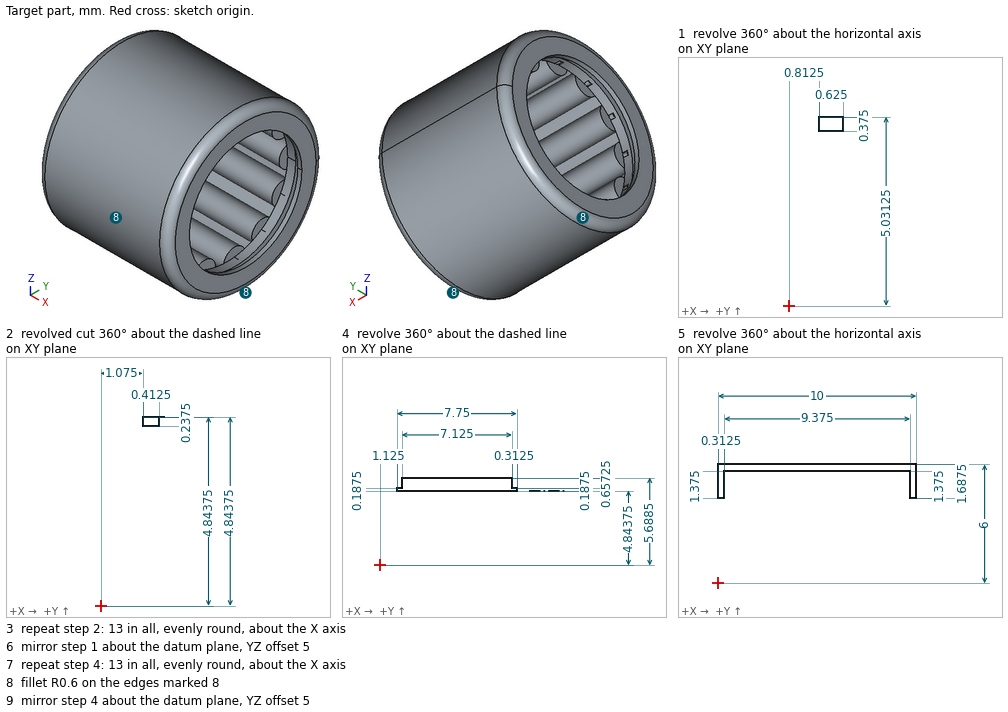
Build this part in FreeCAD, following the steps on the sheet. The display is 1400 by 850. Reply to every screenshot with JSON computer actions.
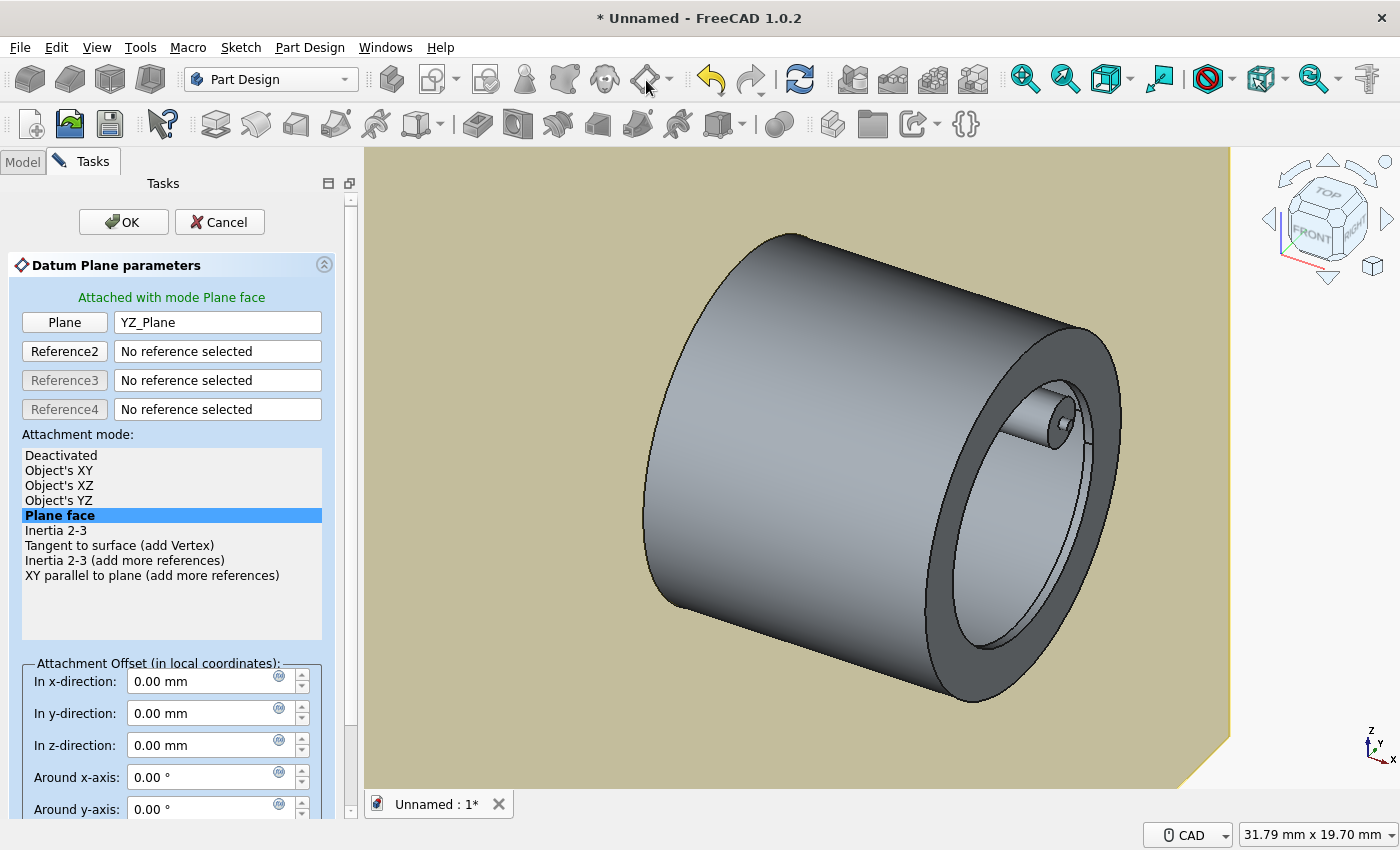
{"action": "triple_click", "coordinate": [210, 745]}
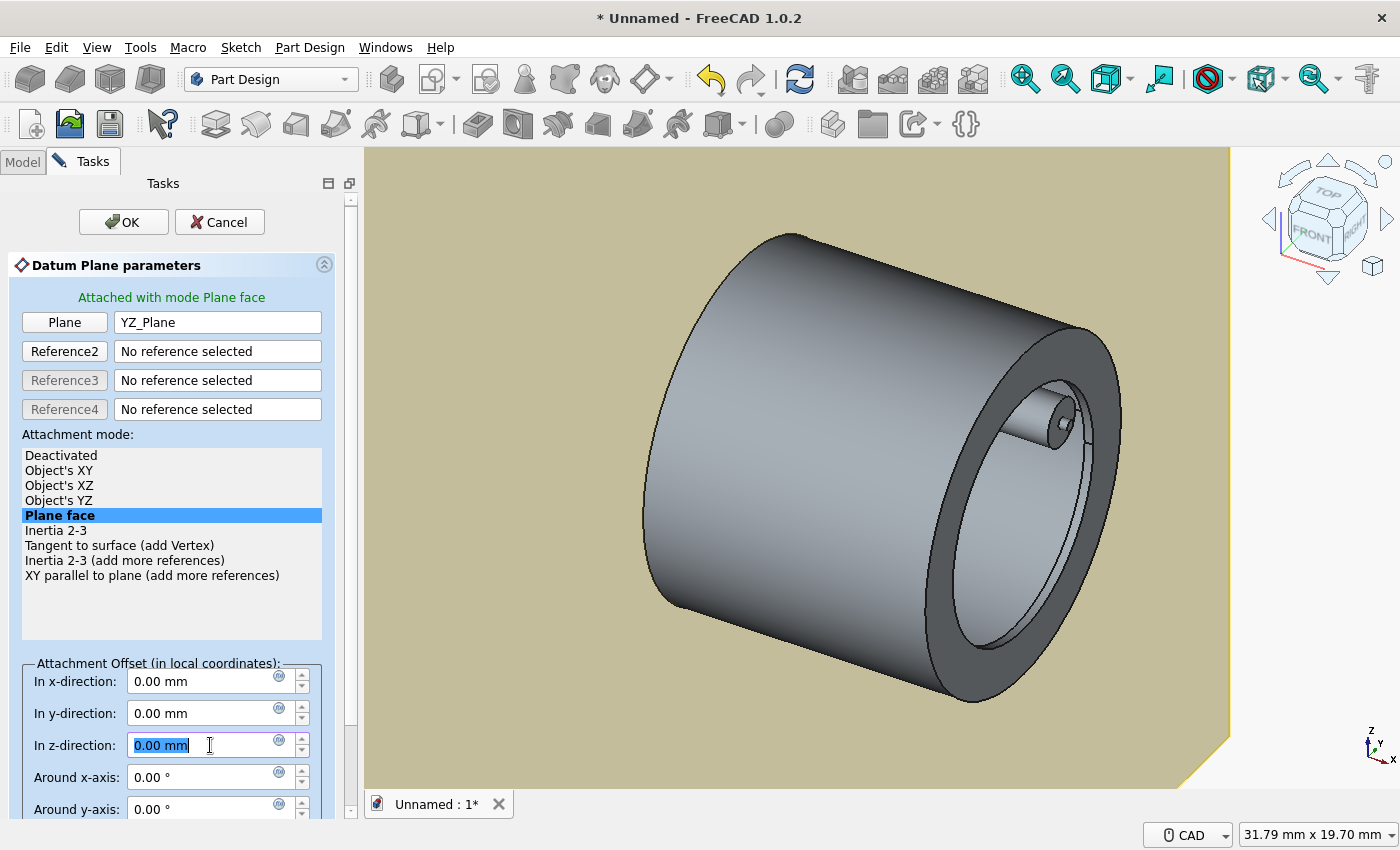
{"action": "type", "text": "5"}
{"action": "key", "text": "Tab"}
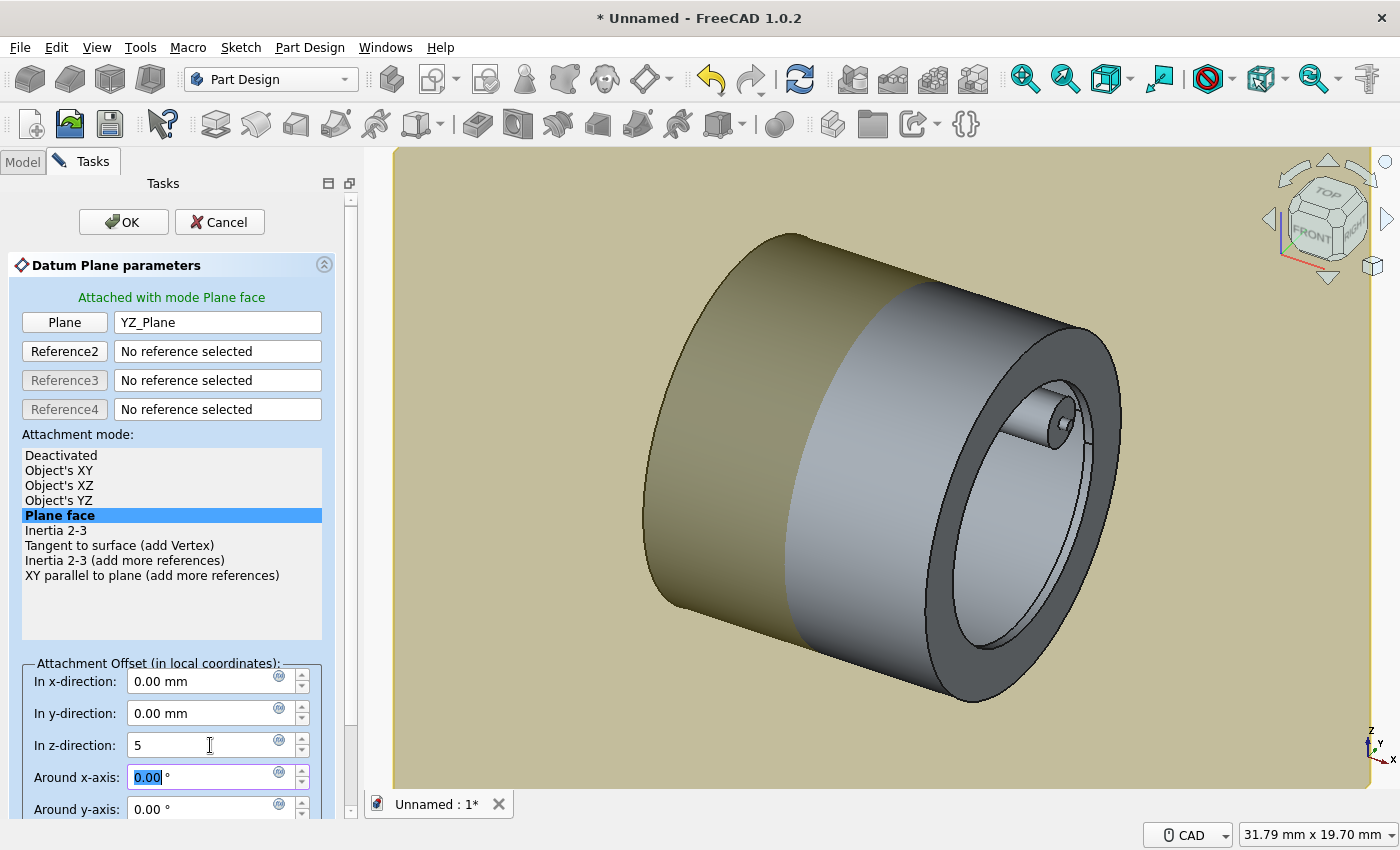
{"action": "left_click", "coordinate": [124, 222]}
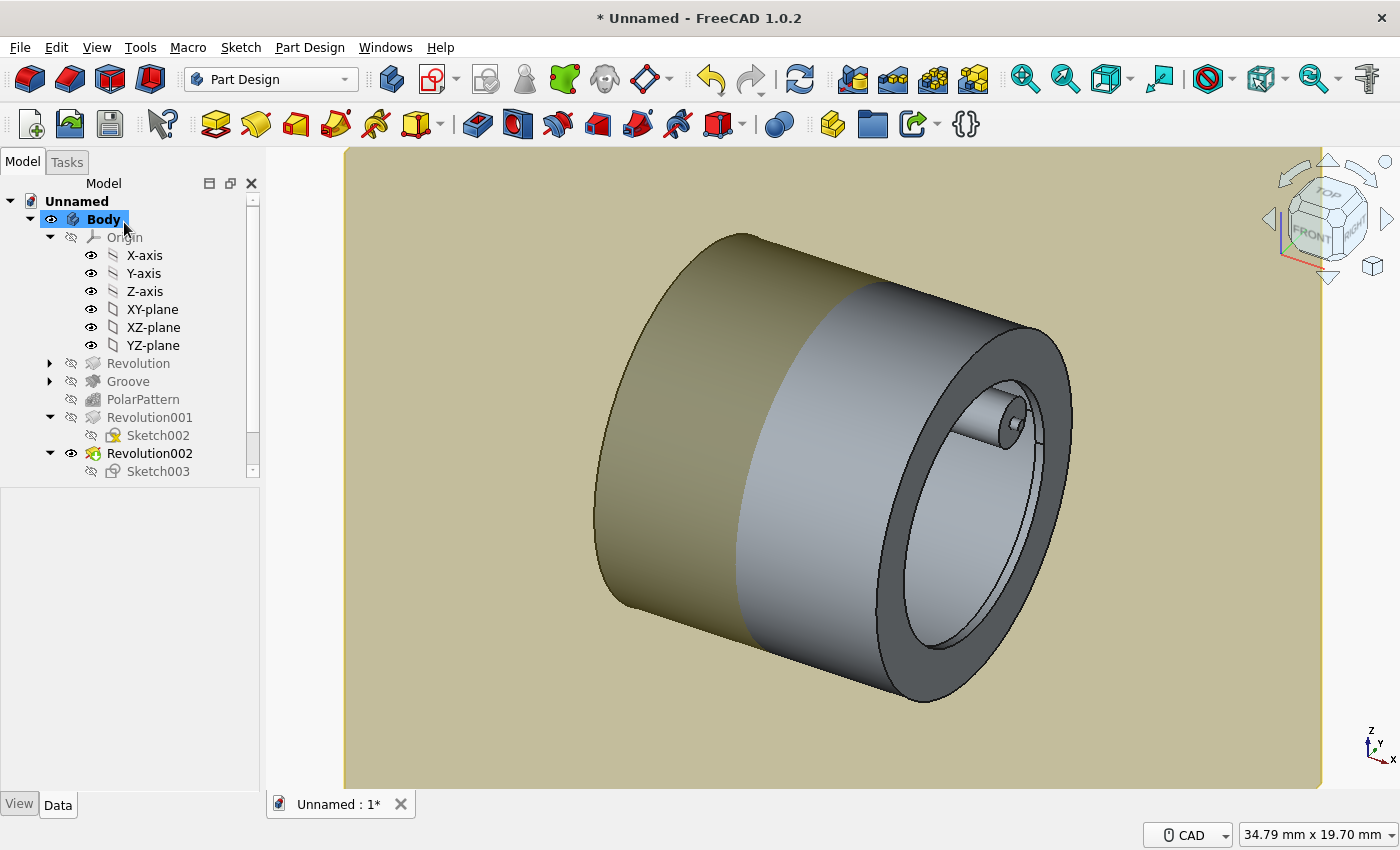
{"action": "left_click", "coordinate": [116, 363]}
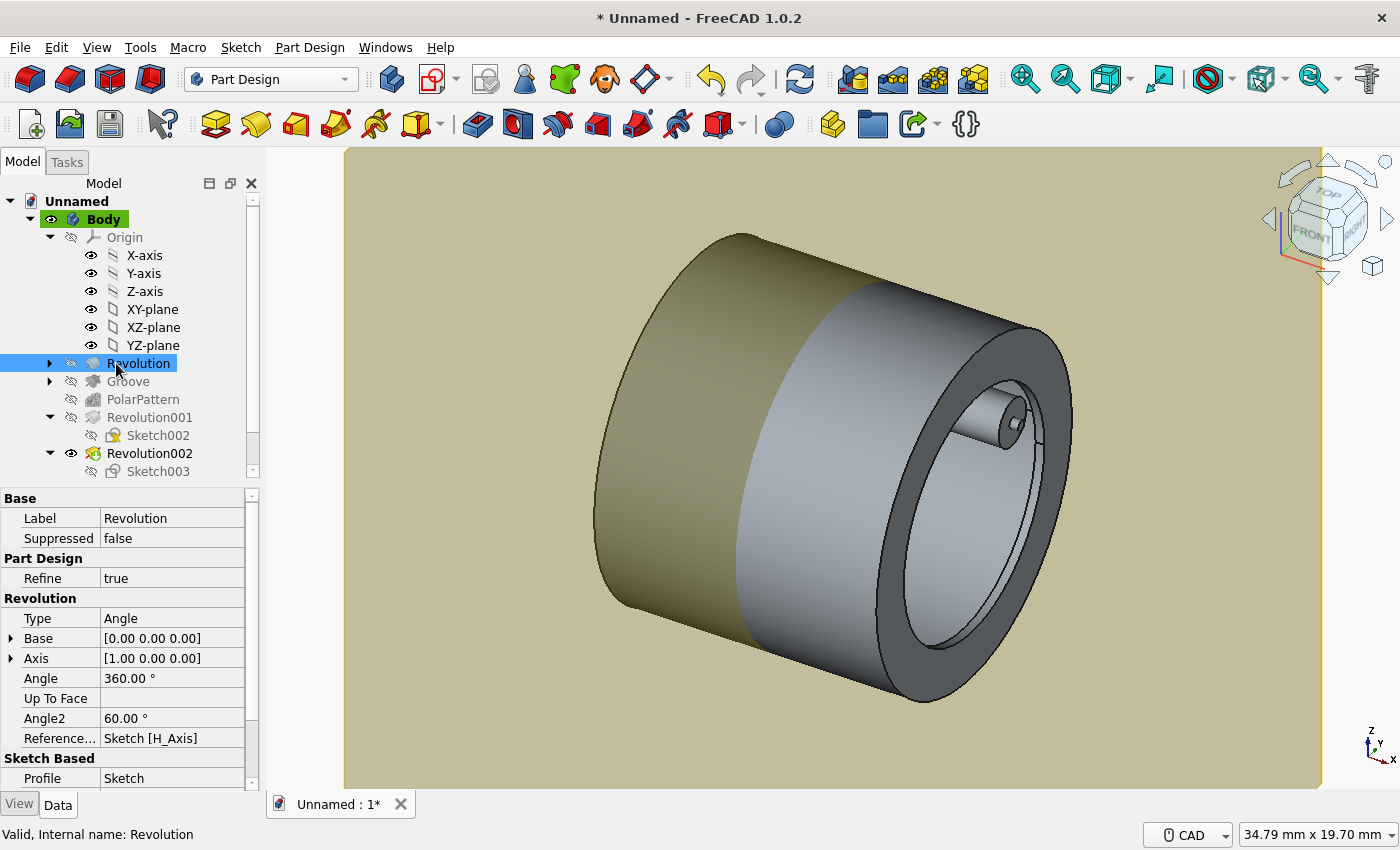
{"action": "left_click", "coordinate": [854, 80]}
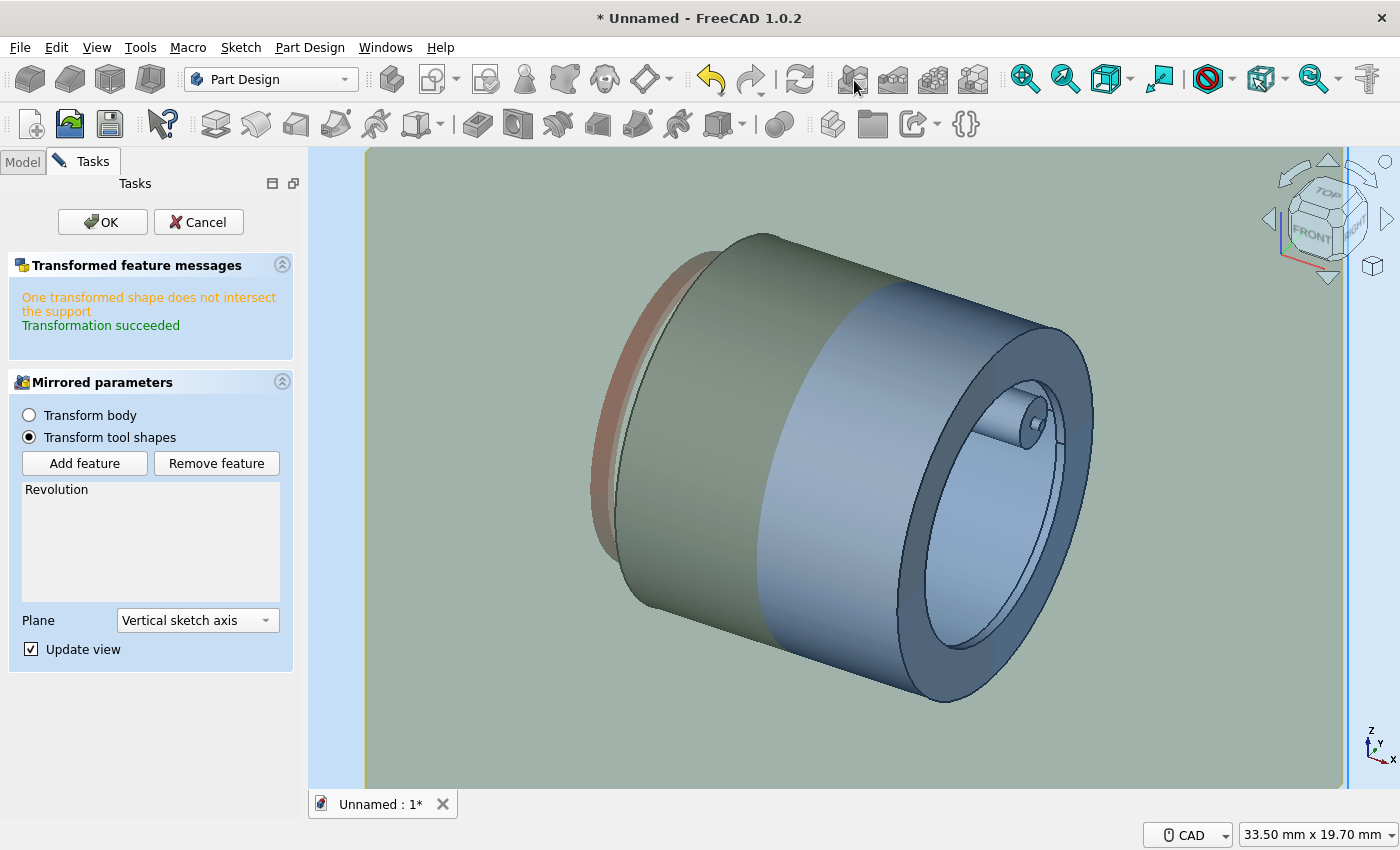
{"action": "left_click", "coordinate": [198, 620]}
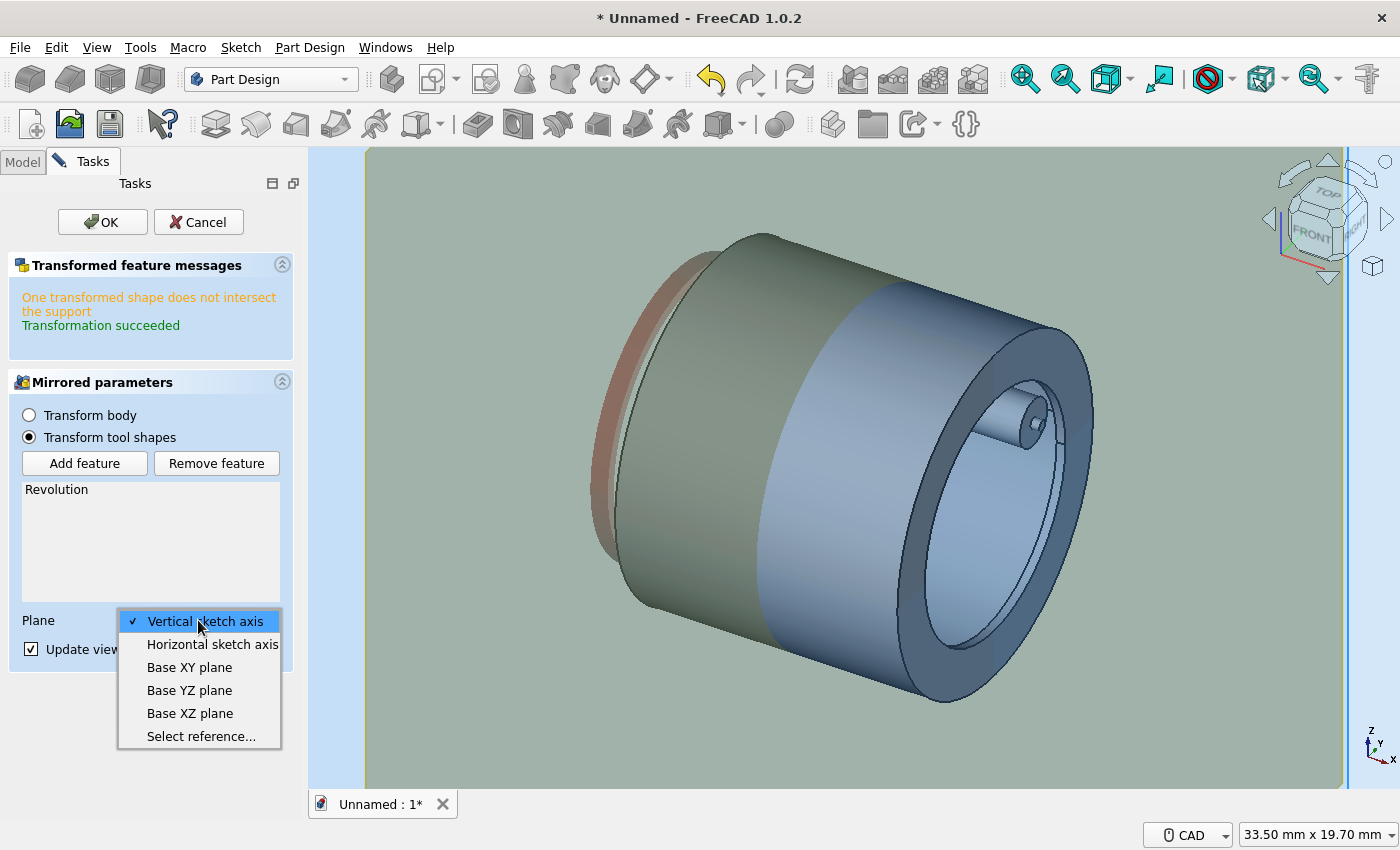
{"action": "left_click", "coordinate": [198, 736]}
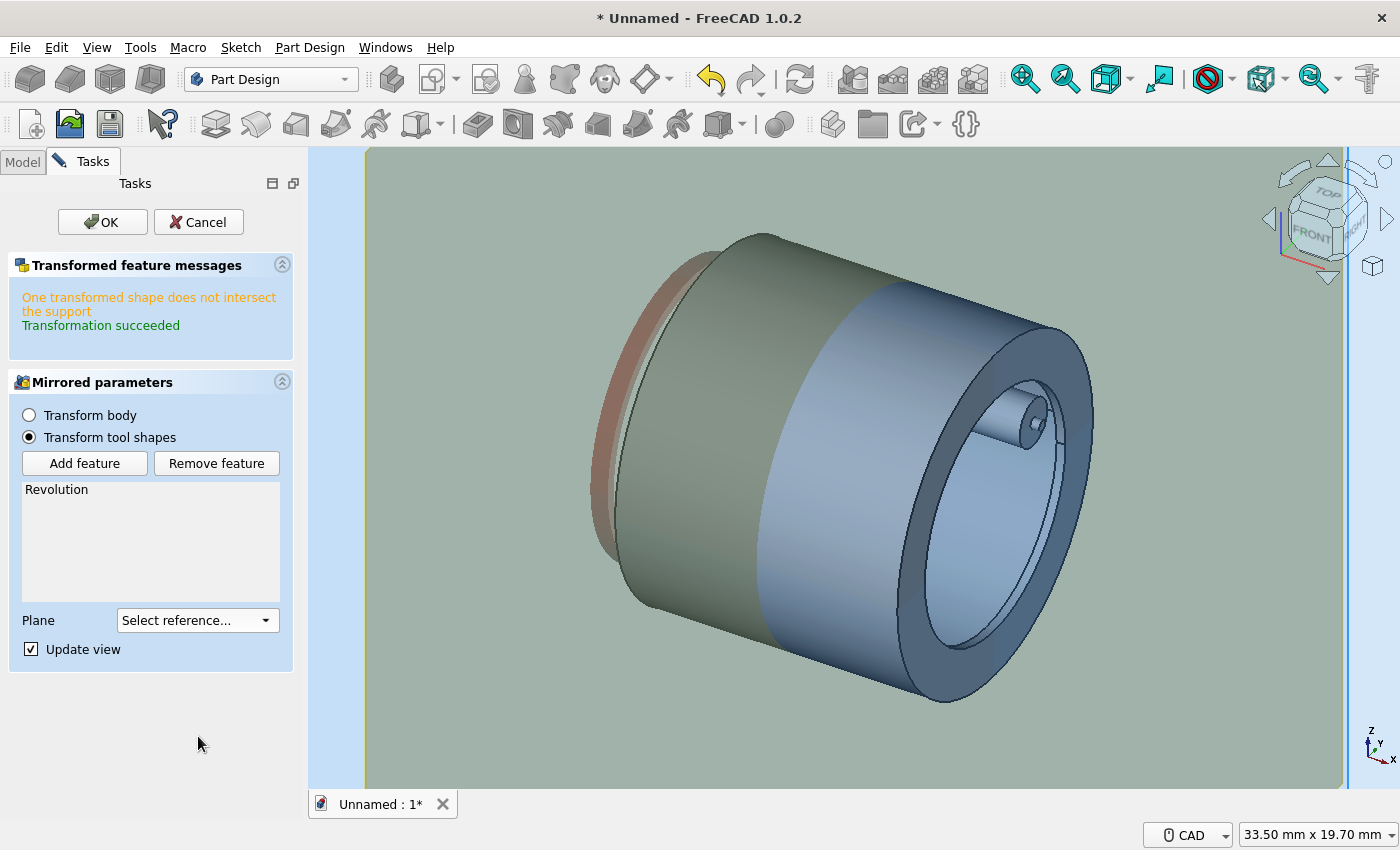
{"action": "left_click", "coordinate": [23, 161]}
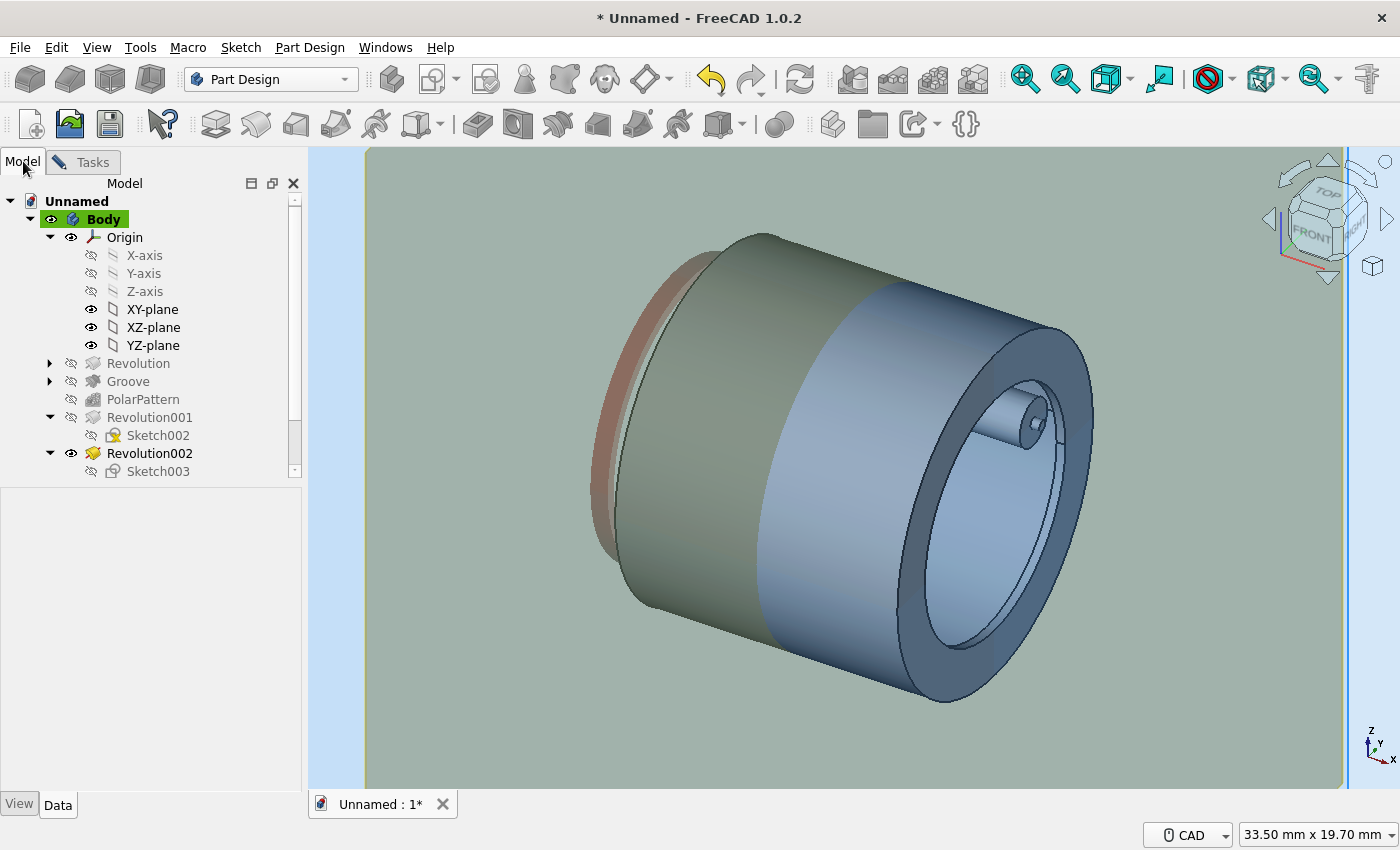
{"action": "scroll", "coordinate": [100, 341], "scroll_direction": "down", "scroll_amount": 3}